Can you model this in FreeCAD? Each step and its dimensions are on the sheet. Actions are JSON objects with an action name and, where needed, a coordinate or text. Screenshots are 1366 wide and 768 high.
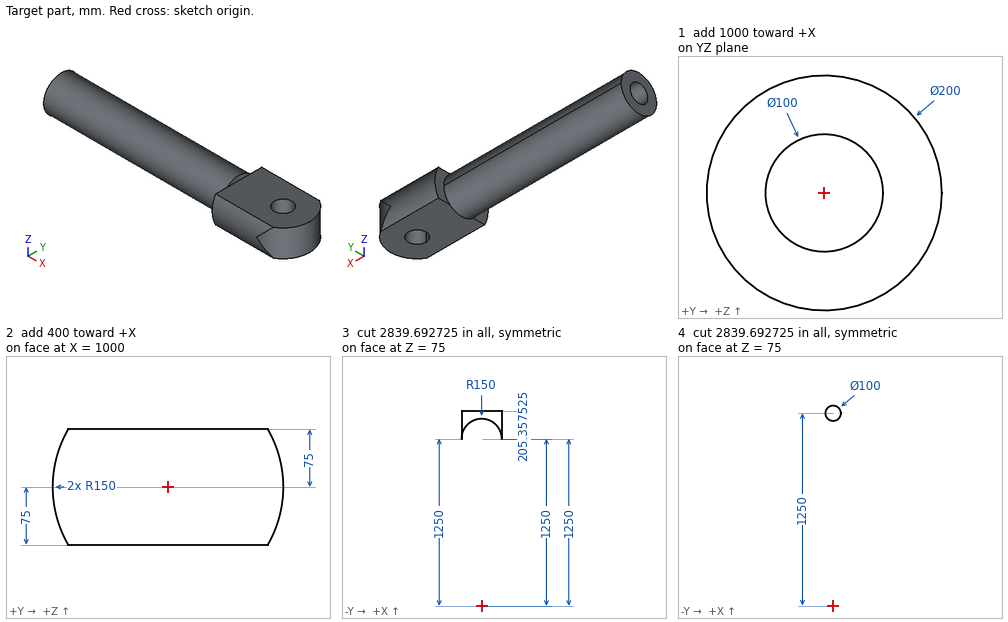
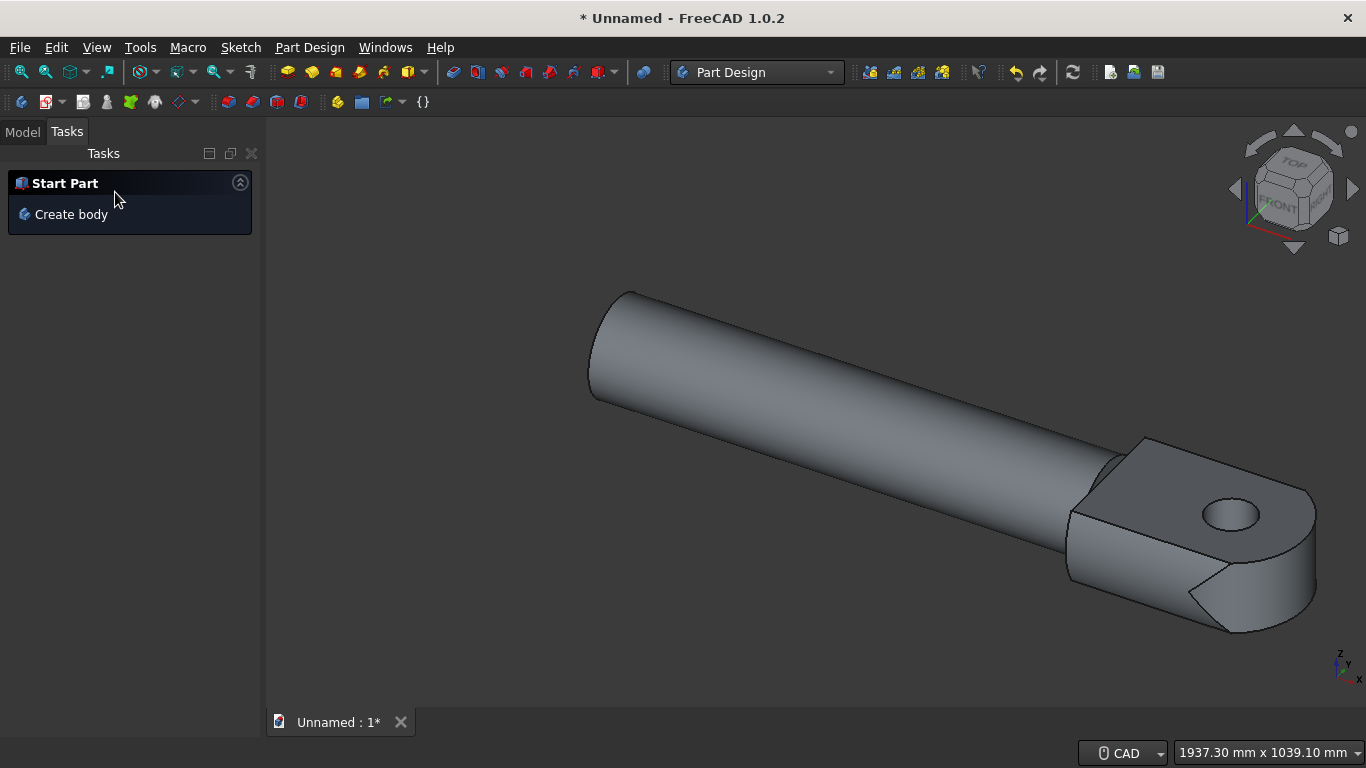
{"action": "key", "text": "0"}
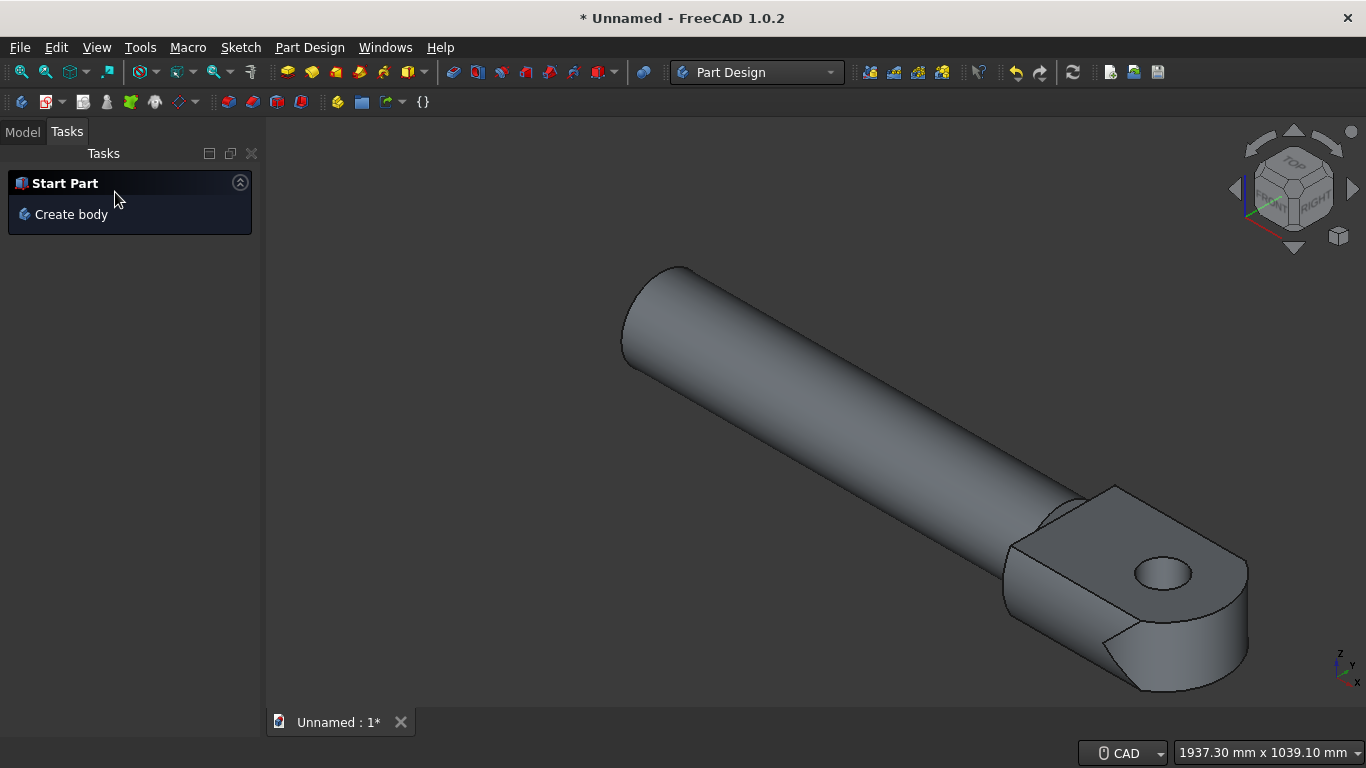
{"action": "left_click", "coordinate": [22, 72]}